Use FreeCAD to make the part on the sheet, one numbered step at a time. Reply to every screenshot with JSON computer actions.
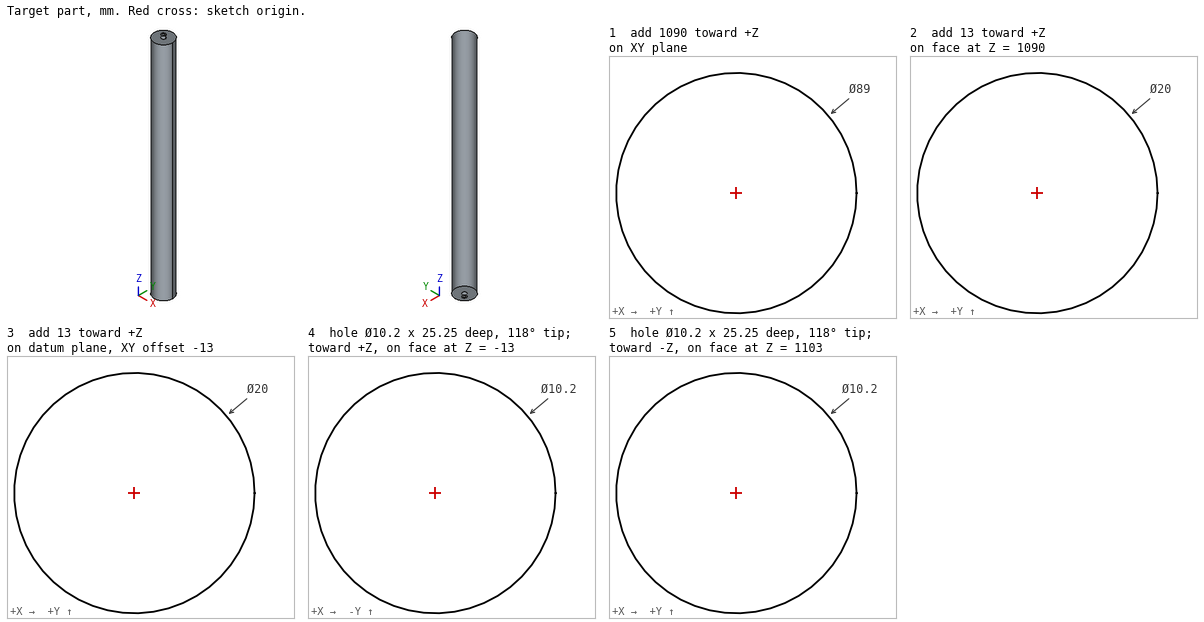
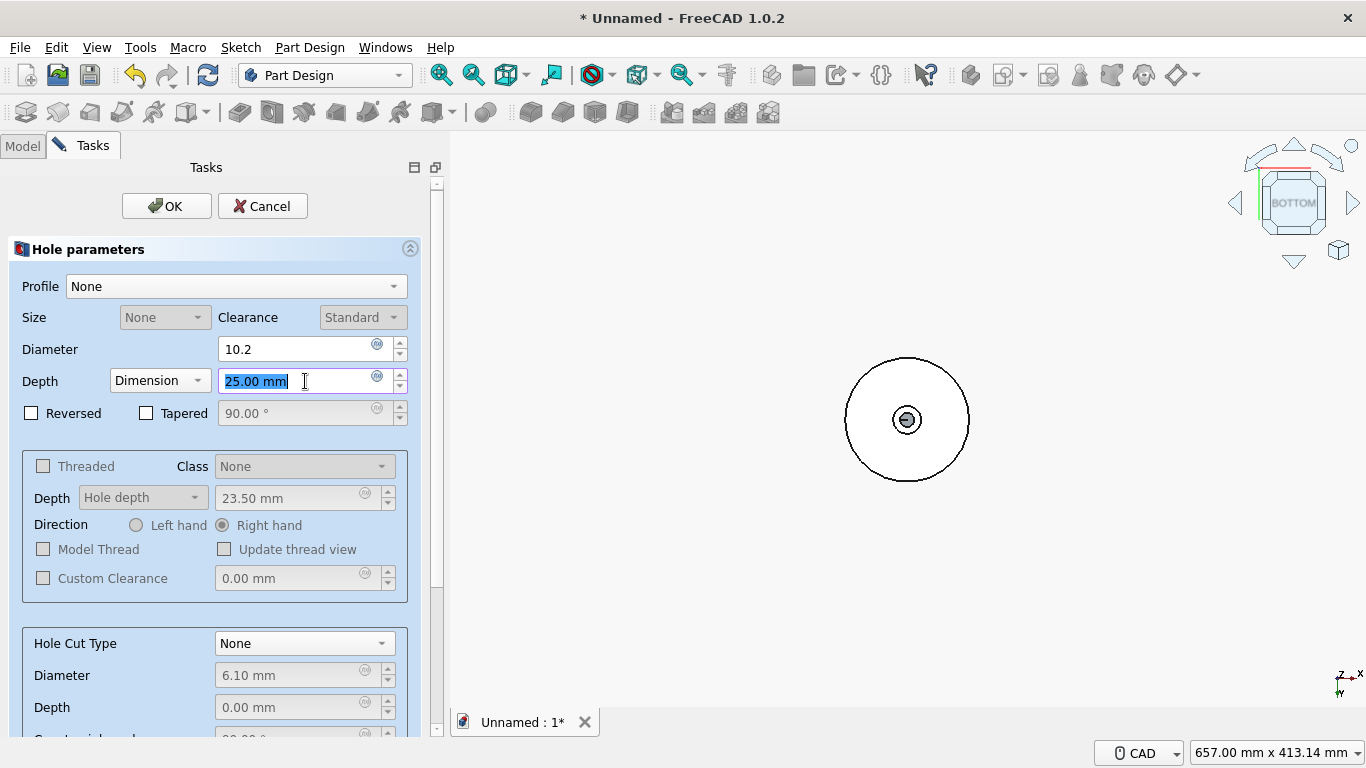
{"action": "type", "text": "25.25"}
{"action": "key", "text": "Tab"}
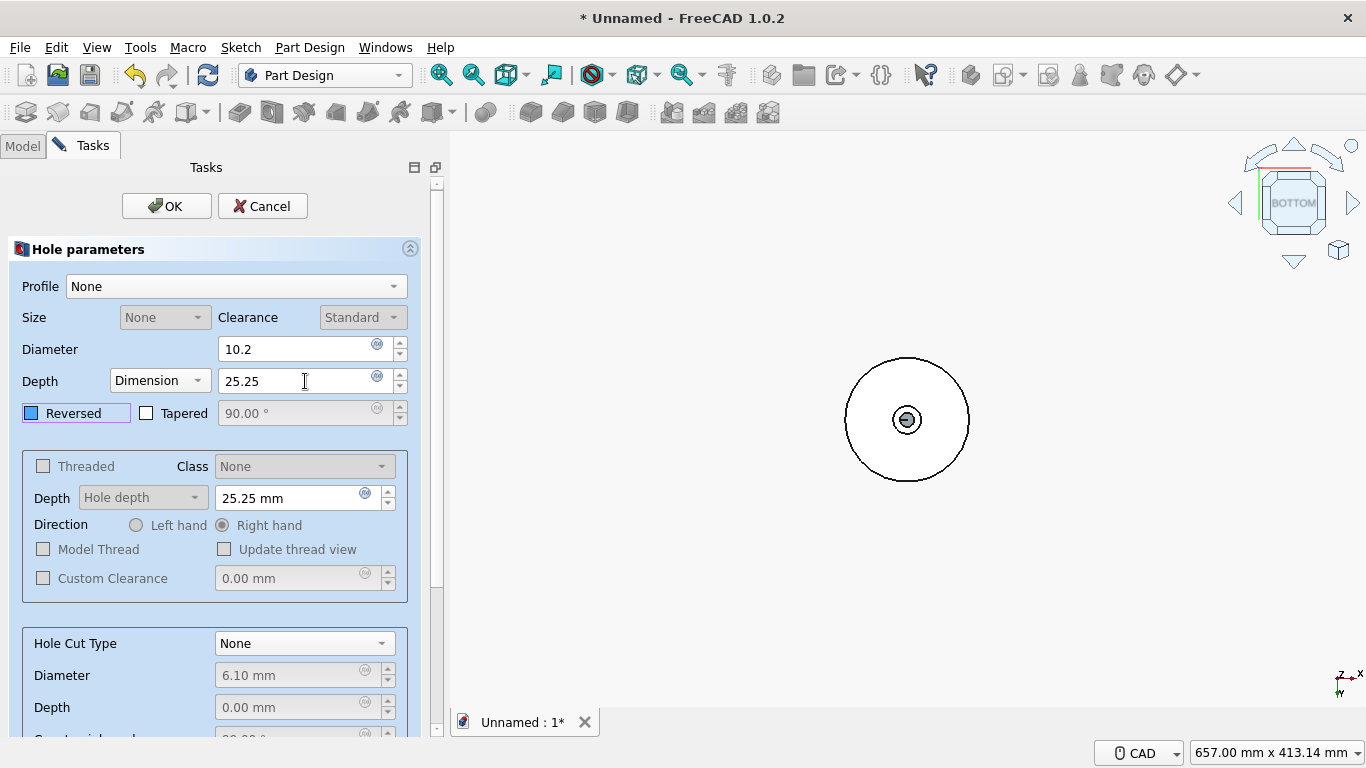
{"action": "left_click", "coordinate": [167, 206]}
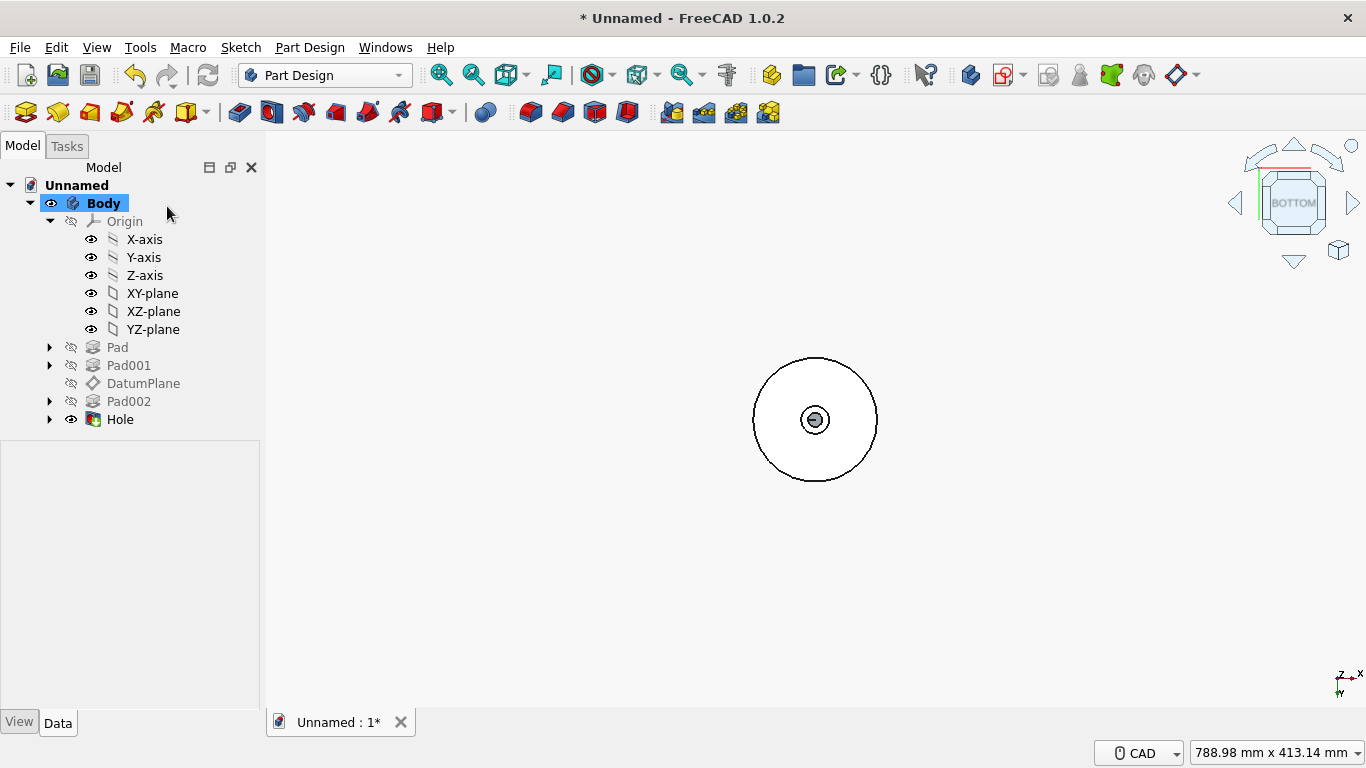
{"action": "left_click", "coordinate": [442, 76]}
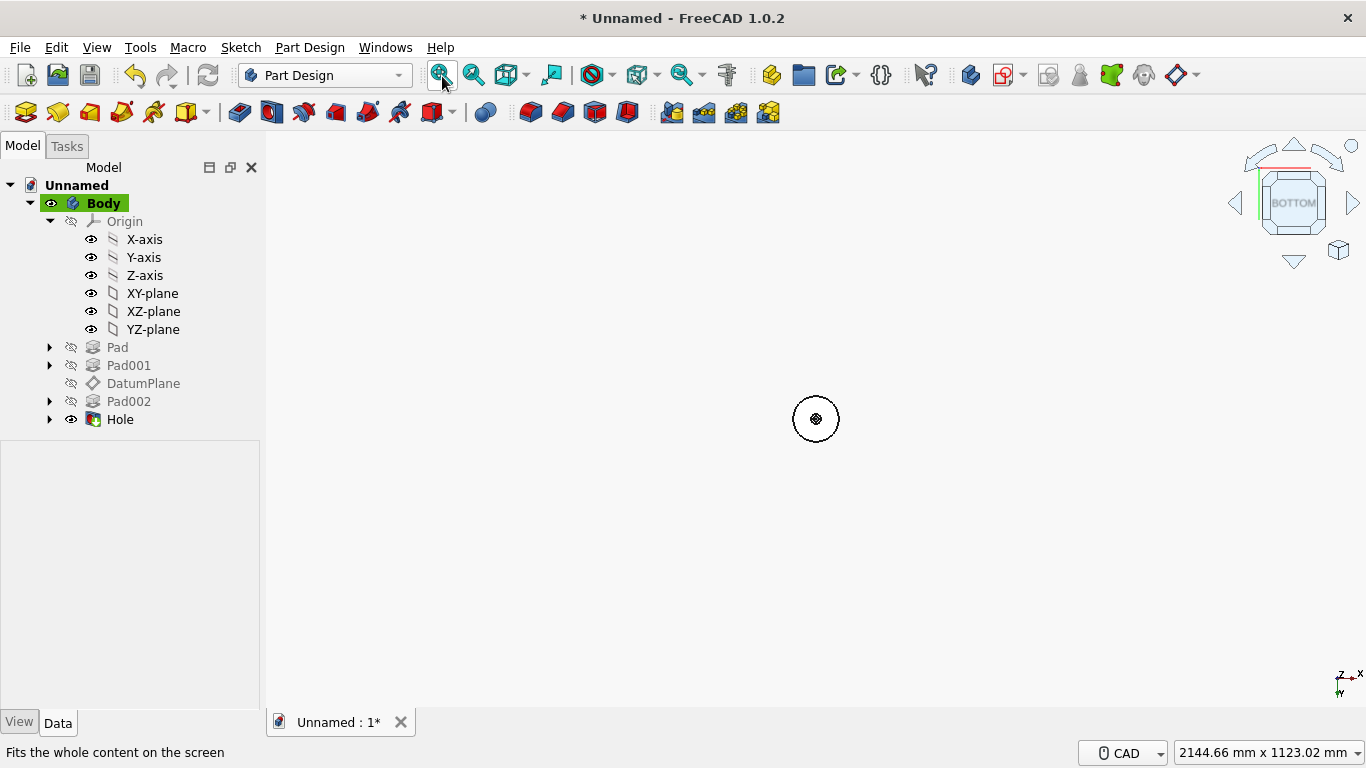
{"action": "key", "text": "0"}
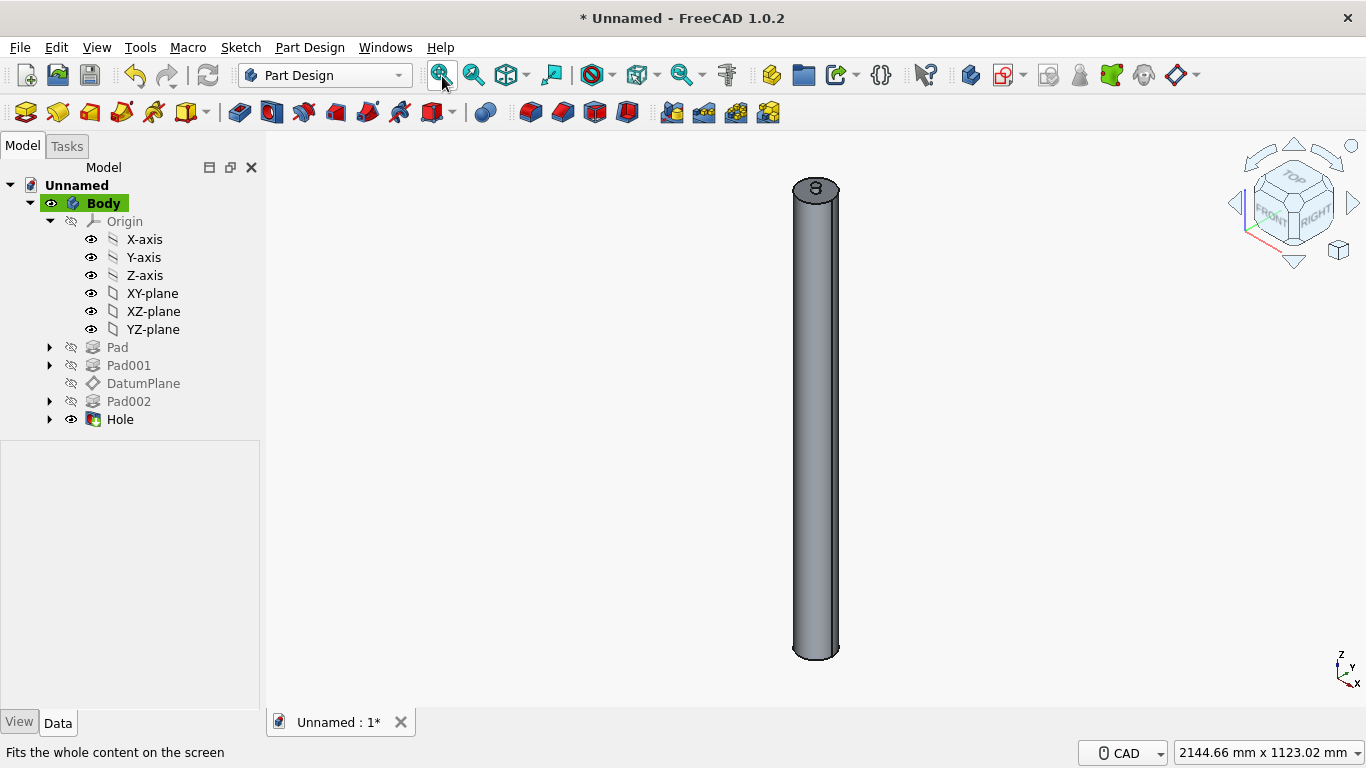
{"action": "scroll", "coordinate": [816, 184], "scroll_direction": "up", "scroll_amount": 5}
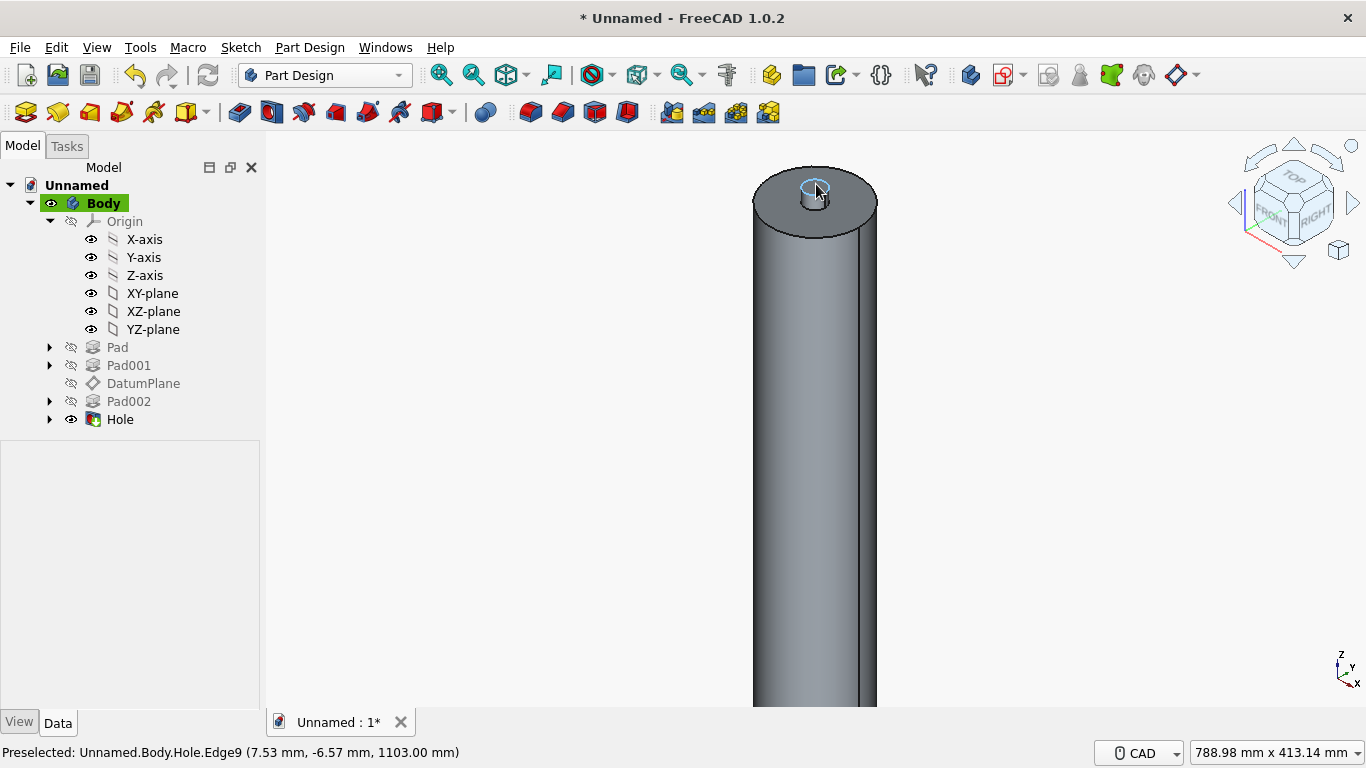
{"action": "left_click", "coordinate": [815, 186]}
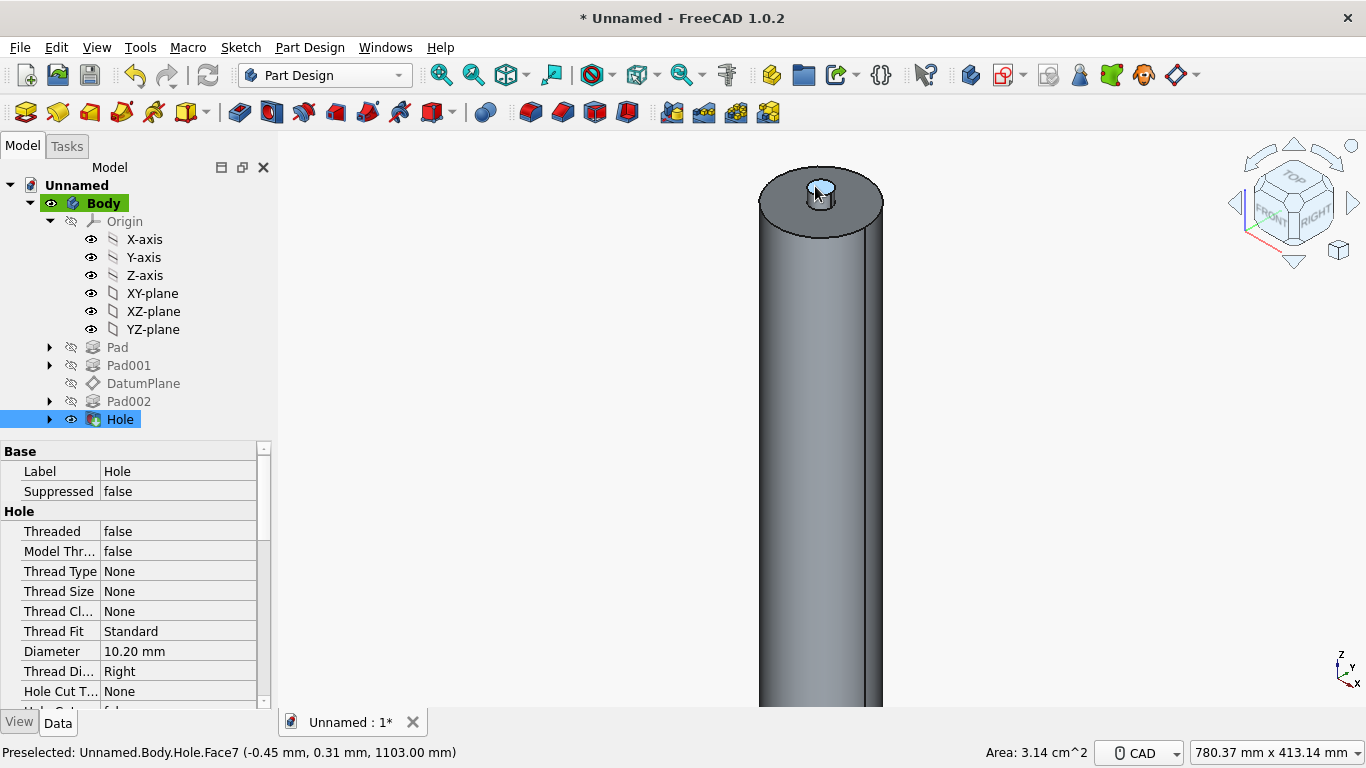
{"action": "left_click", "coordinate": [1004, 76]}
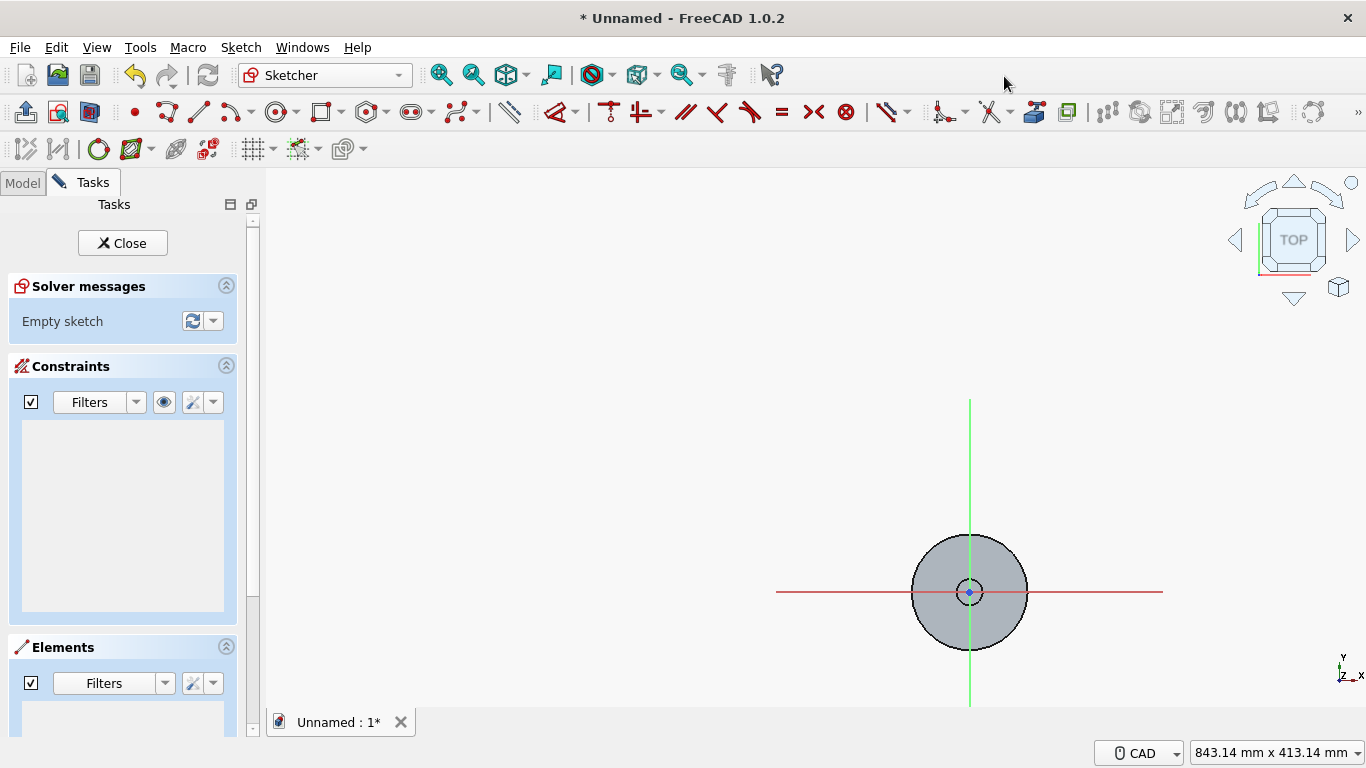
{"action": "scroll", "coordinate": [981, 600], "scroll_direction": "up", "scroll_amount": 15}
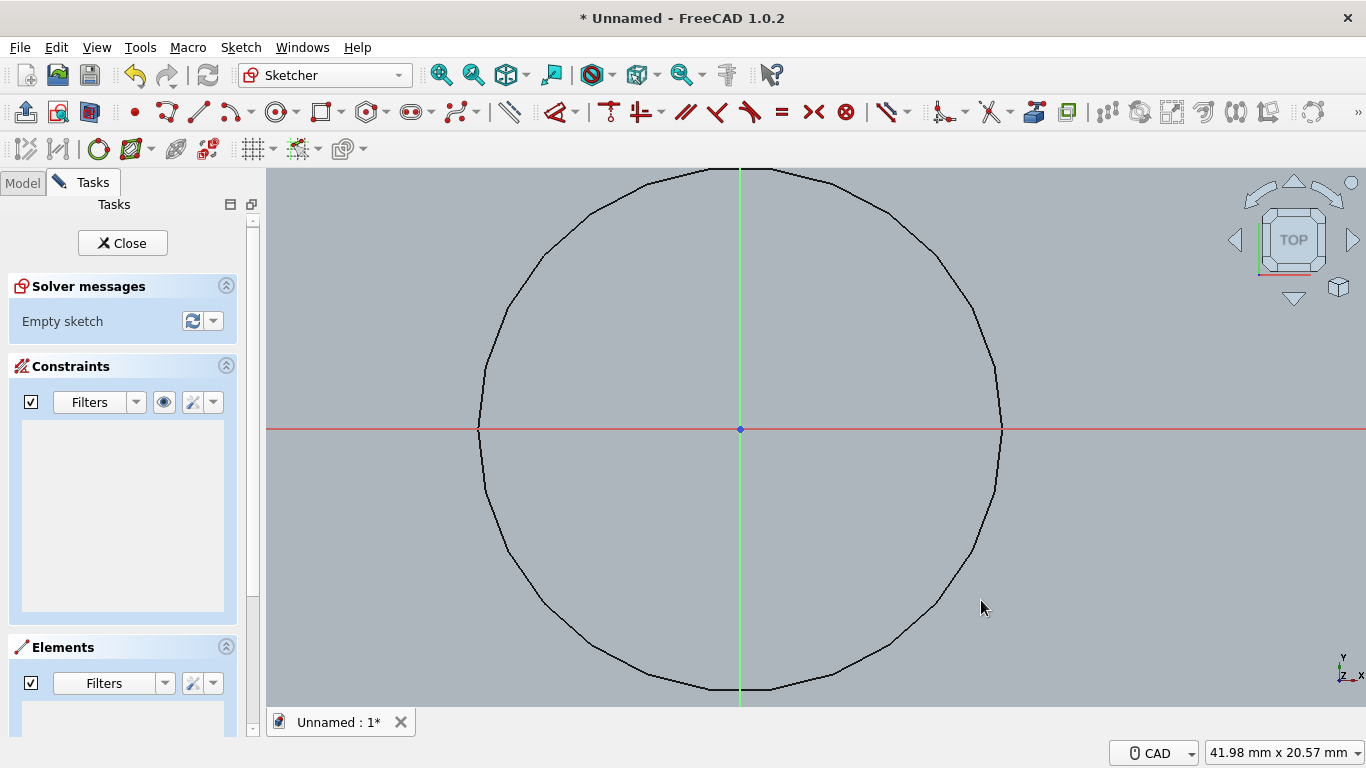
{"action": "left_click", "coordinate": [276, 112]}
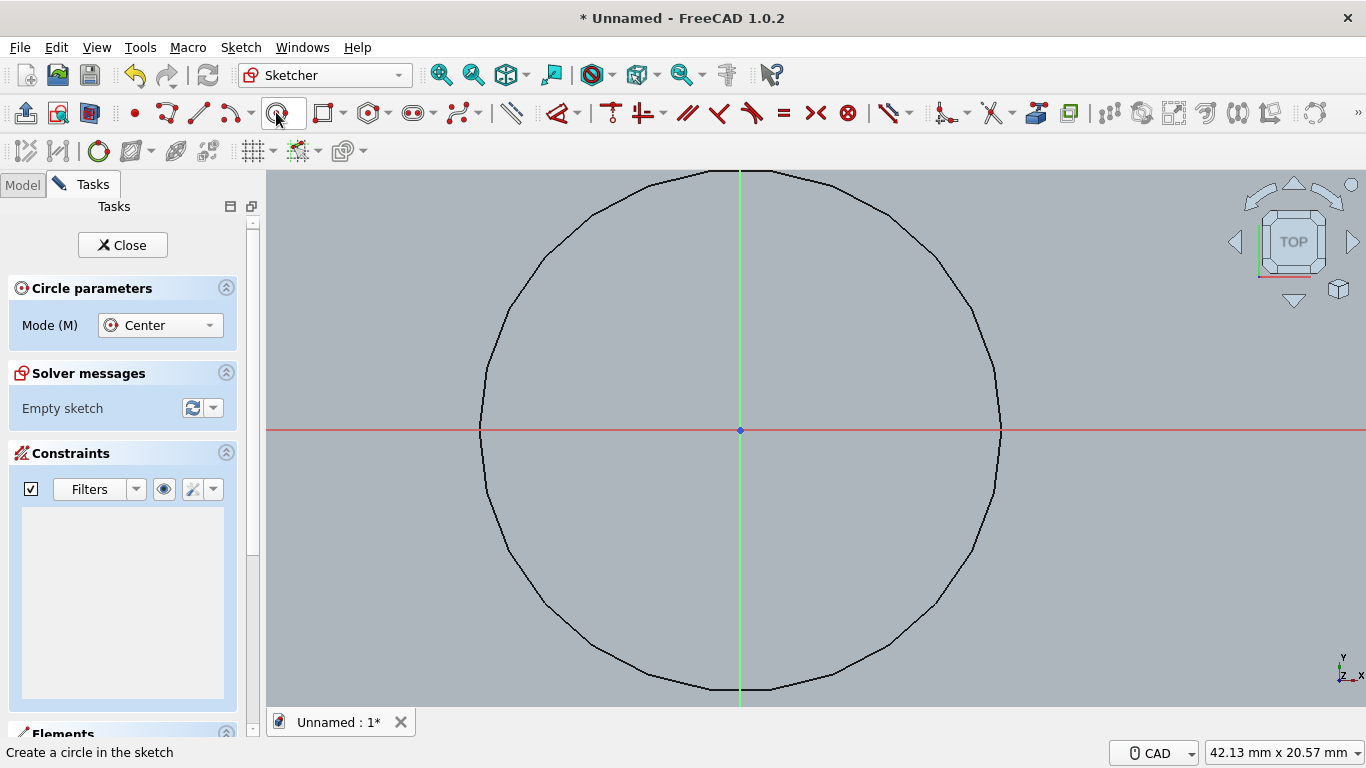
{"action": "left_click", "coordinate": [740, 430]}
{"action": "mouse_move", "coordinate": [835, 336]}